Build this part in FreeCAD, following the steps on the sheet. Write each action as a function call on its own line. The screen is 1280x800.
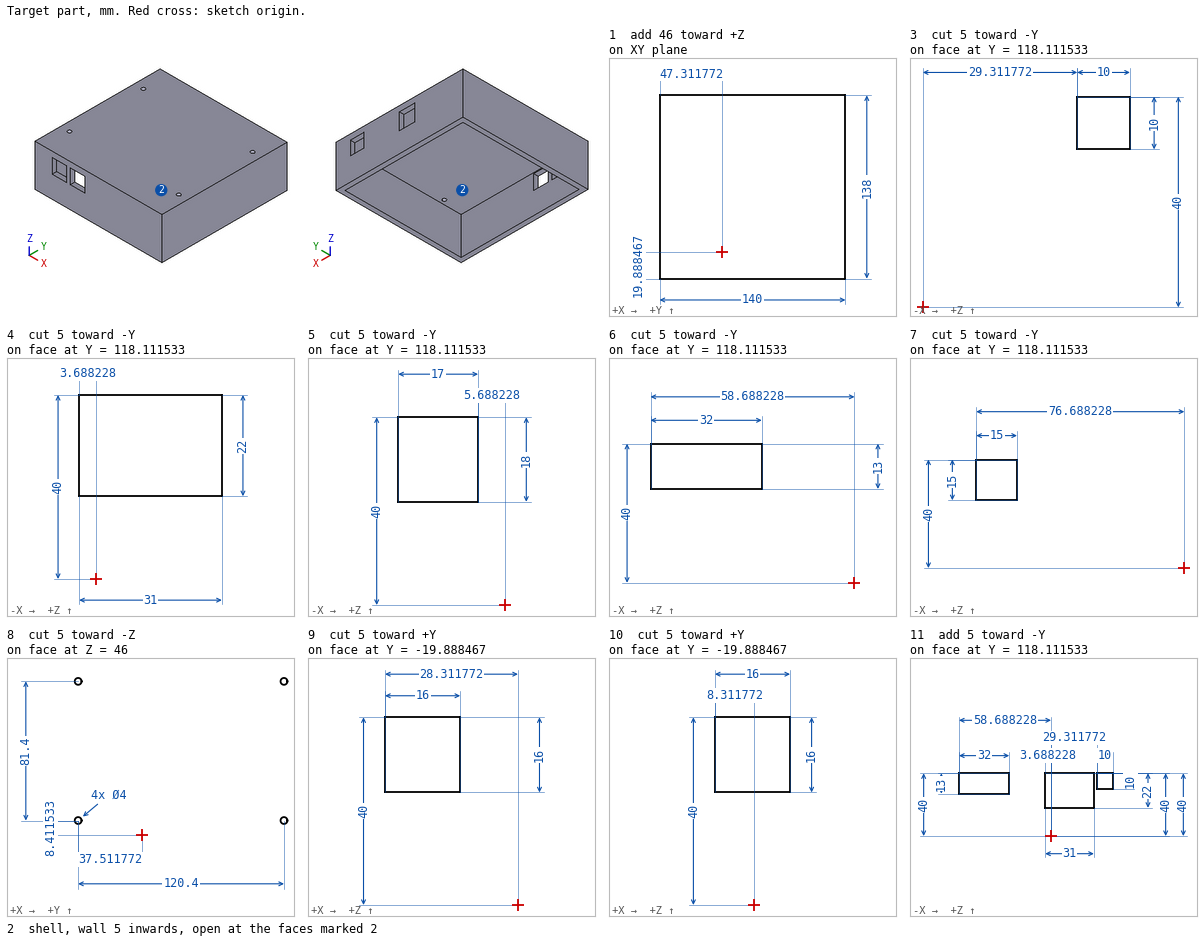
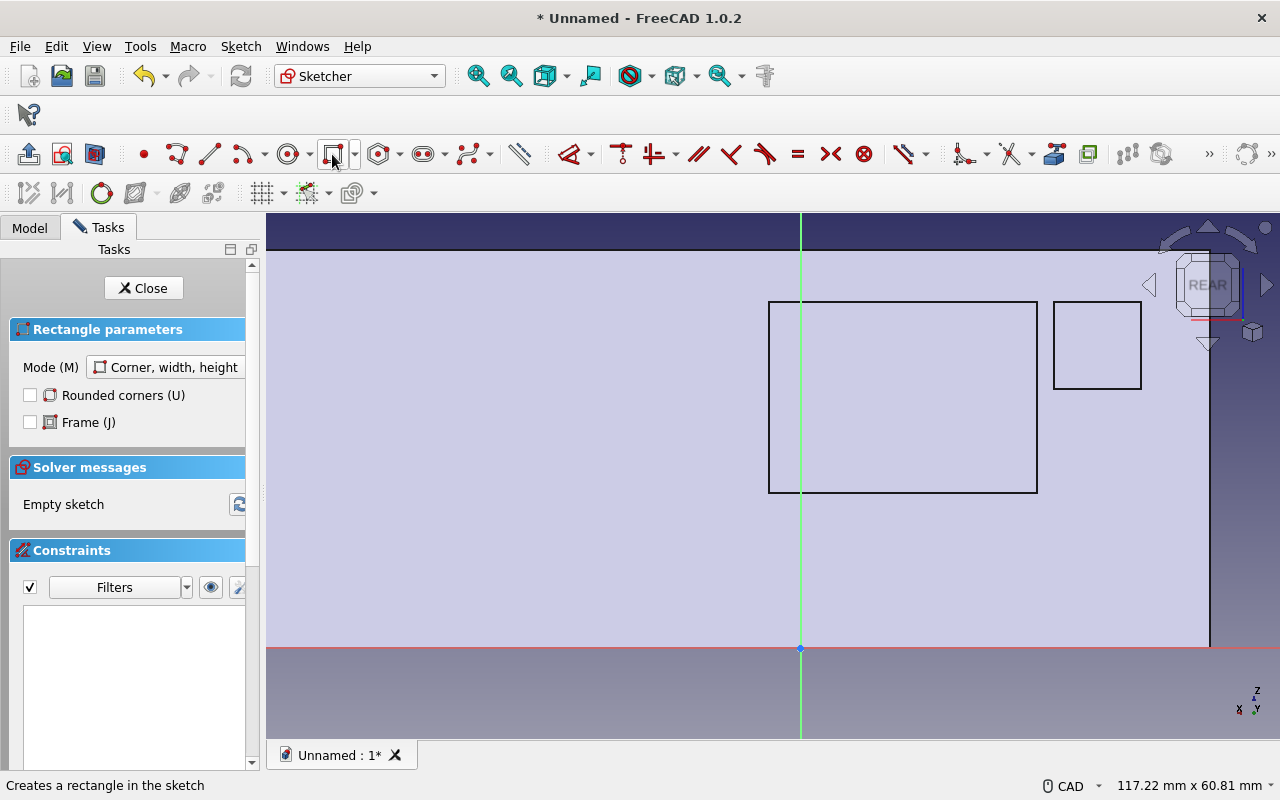
click(605, 302)
move(752, 458)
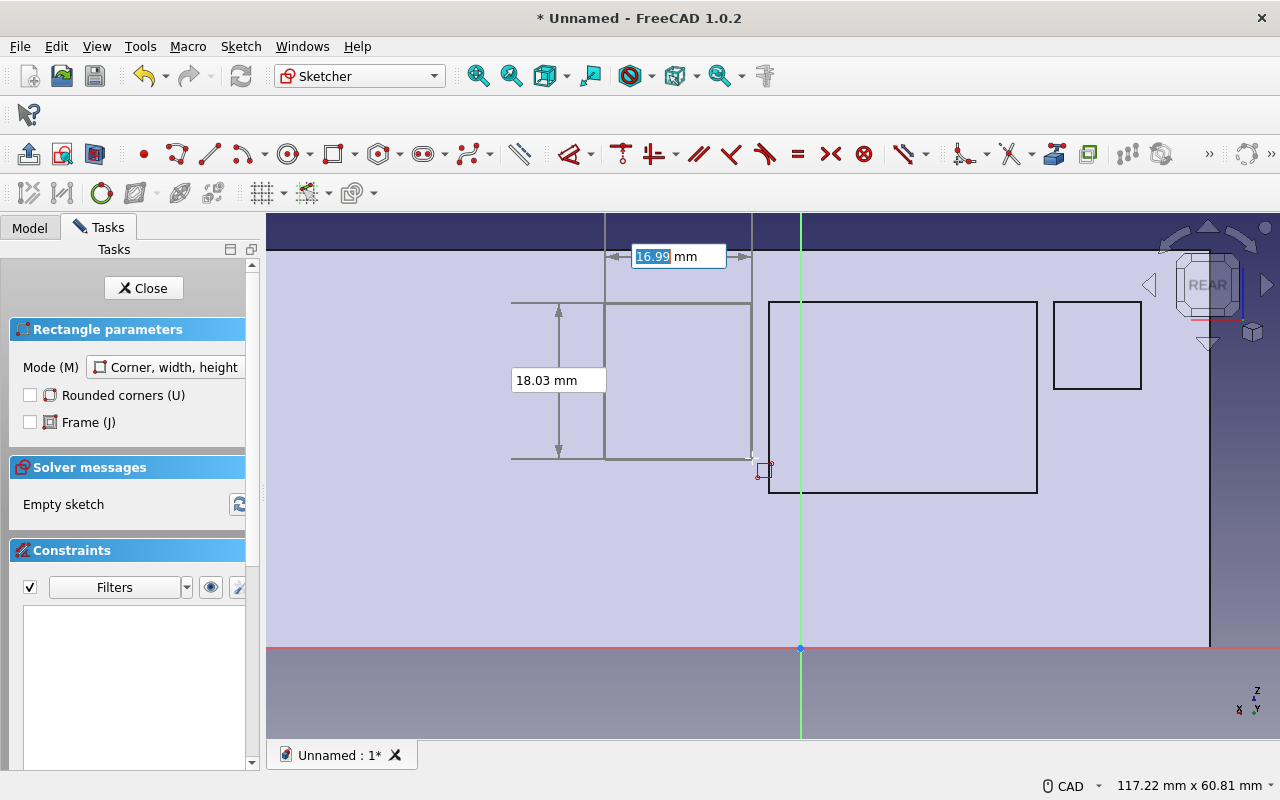
text(17)
key(Tab)
text(18)
key(Return)
key(Escape)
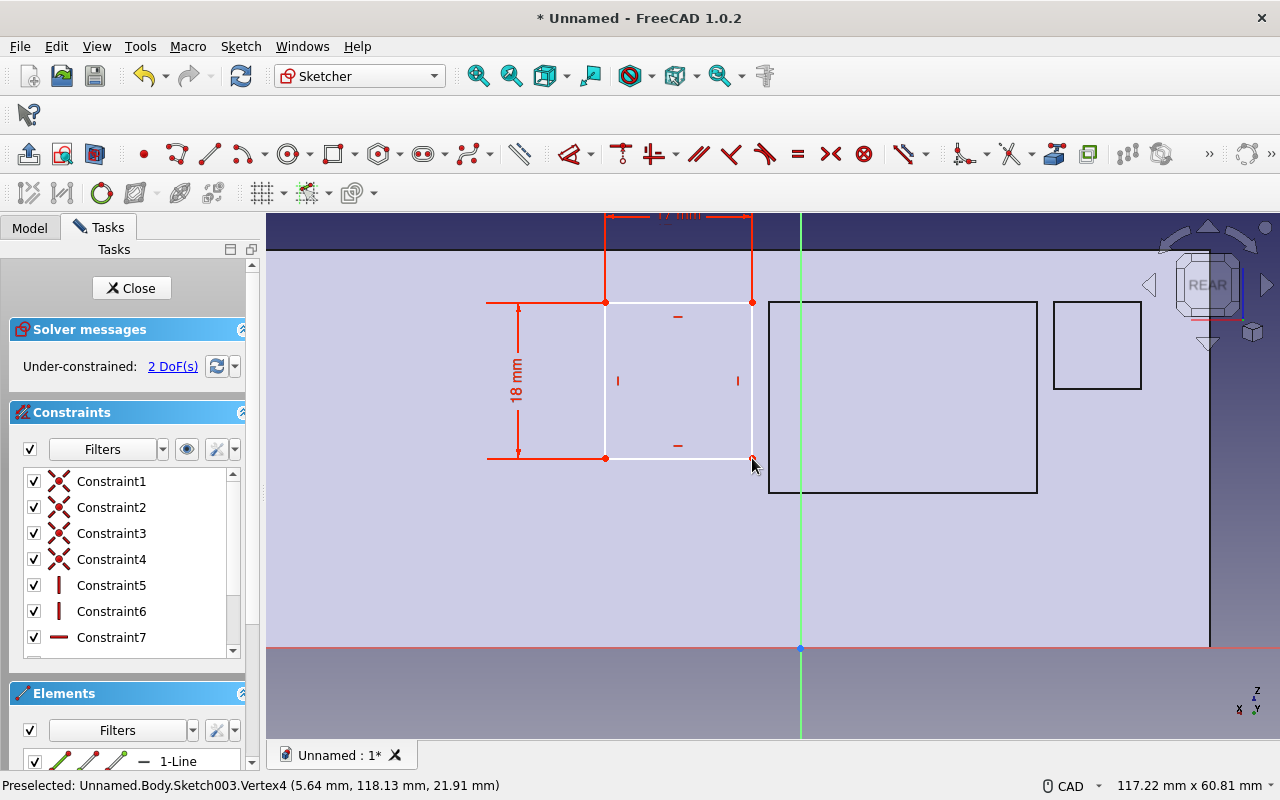
key(d)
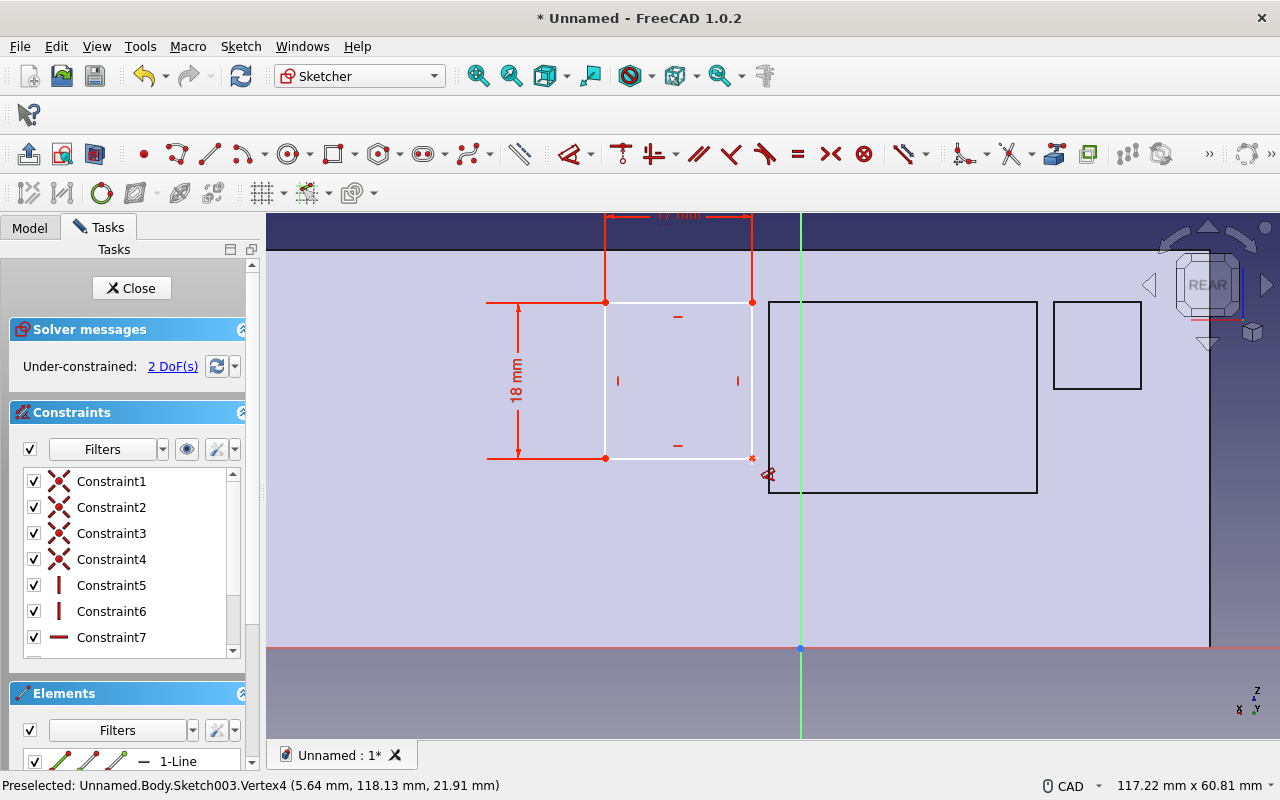
click(605, 303)
click(835, 476)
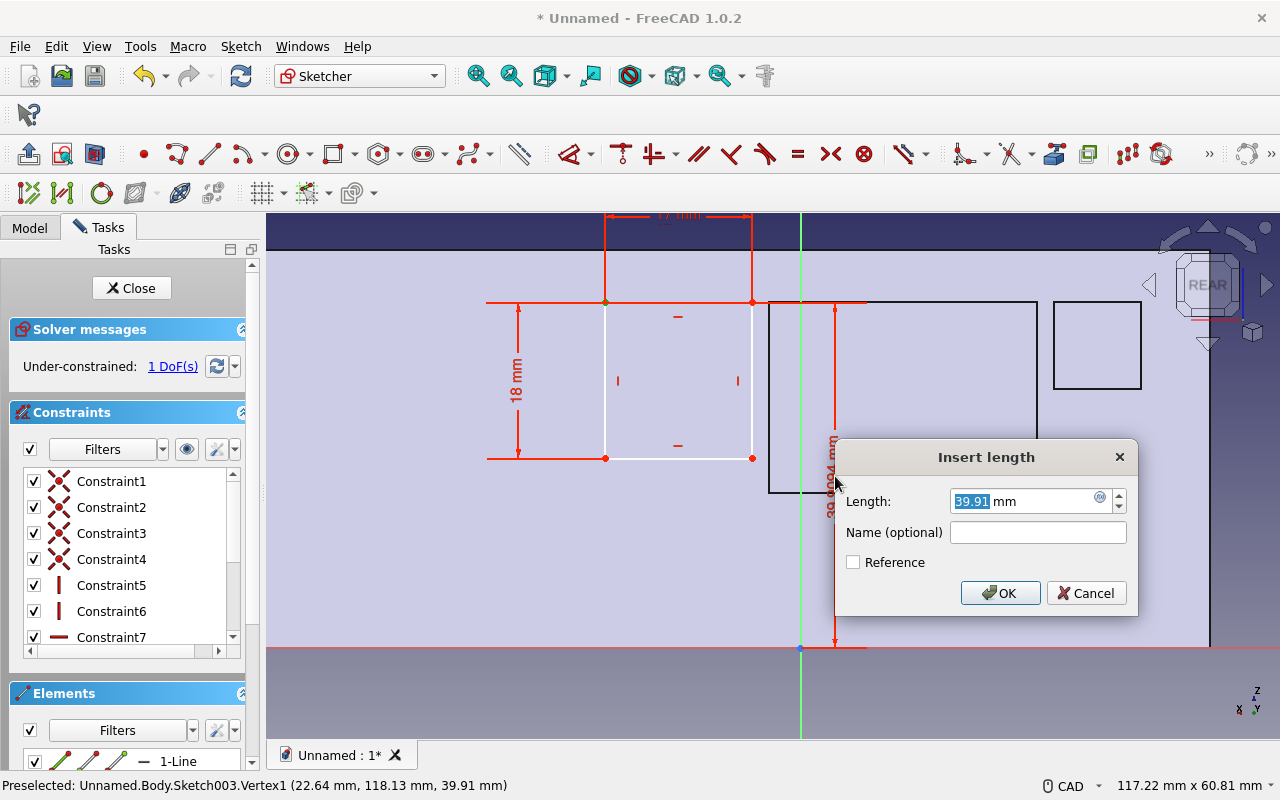
text(40)
key(Return)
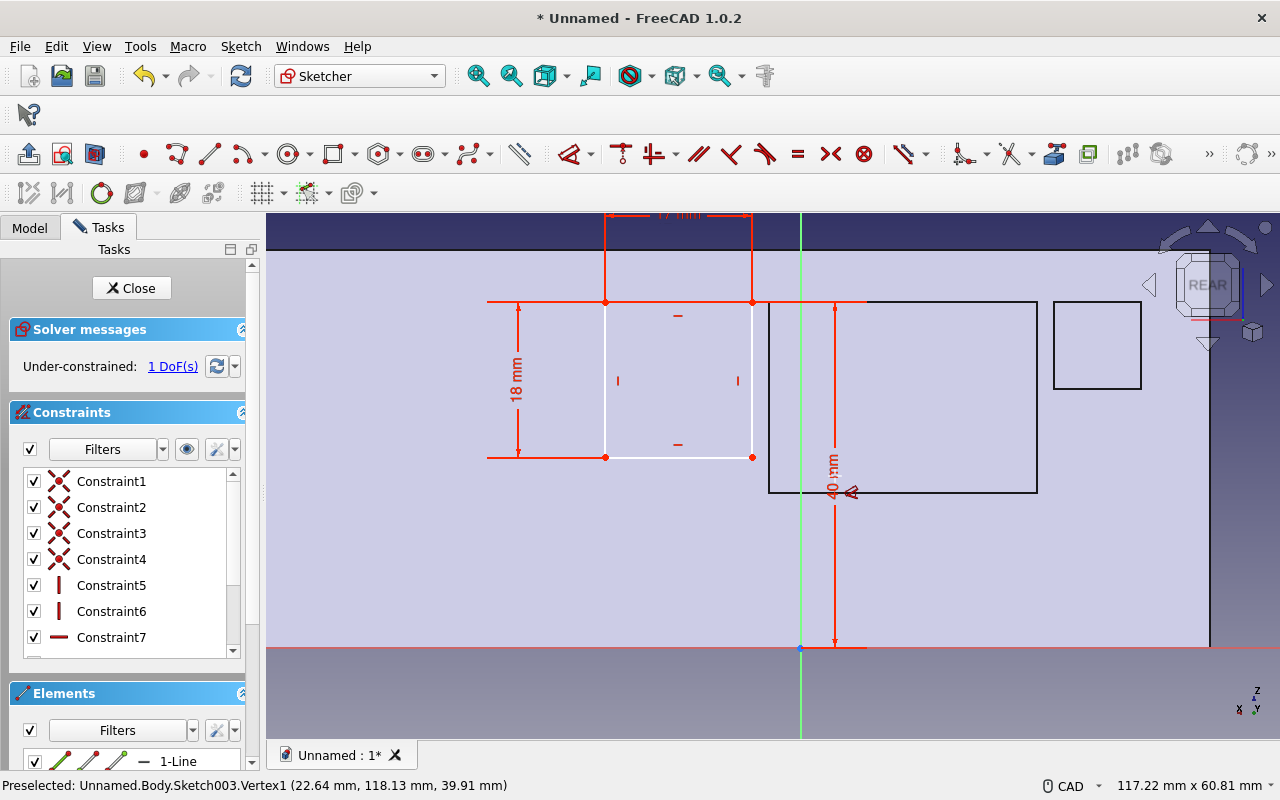
click(752, 458)
click(776, 682)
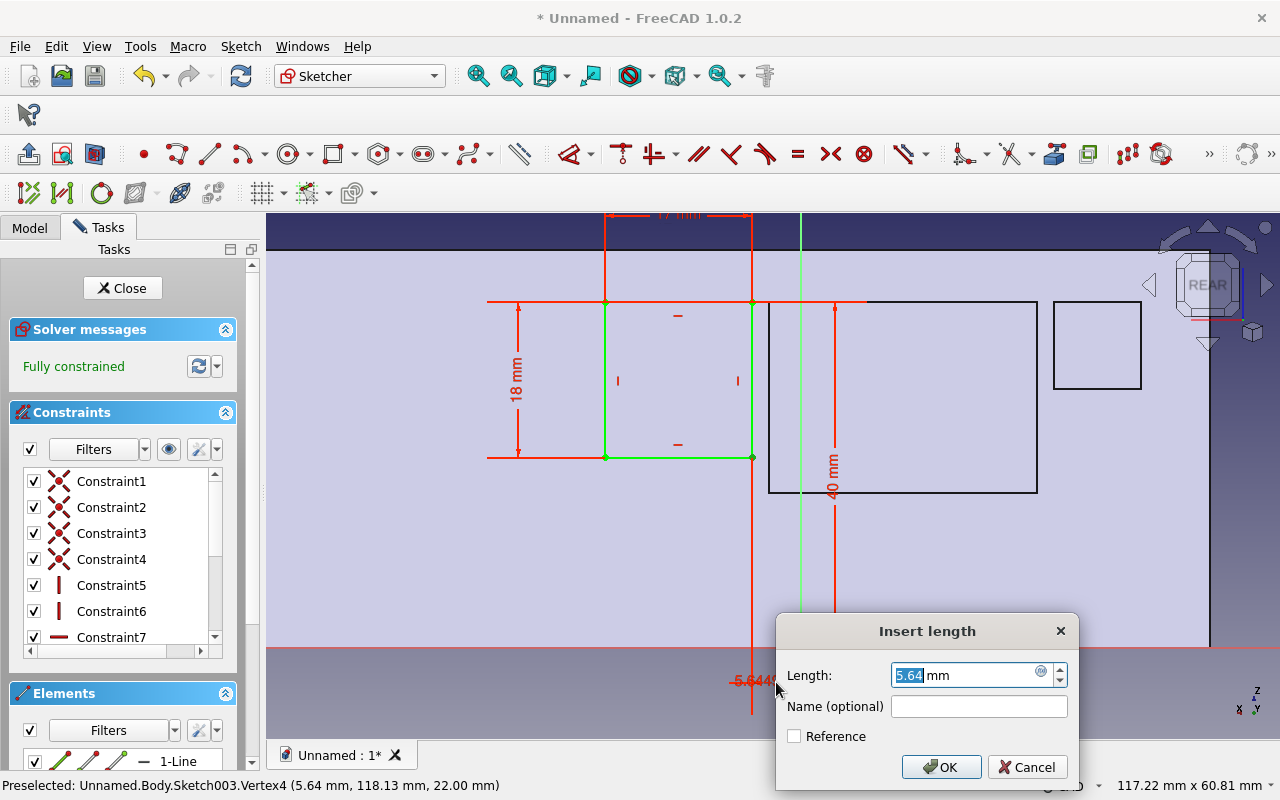
text(5.688228)
key(Return)
key(Escape)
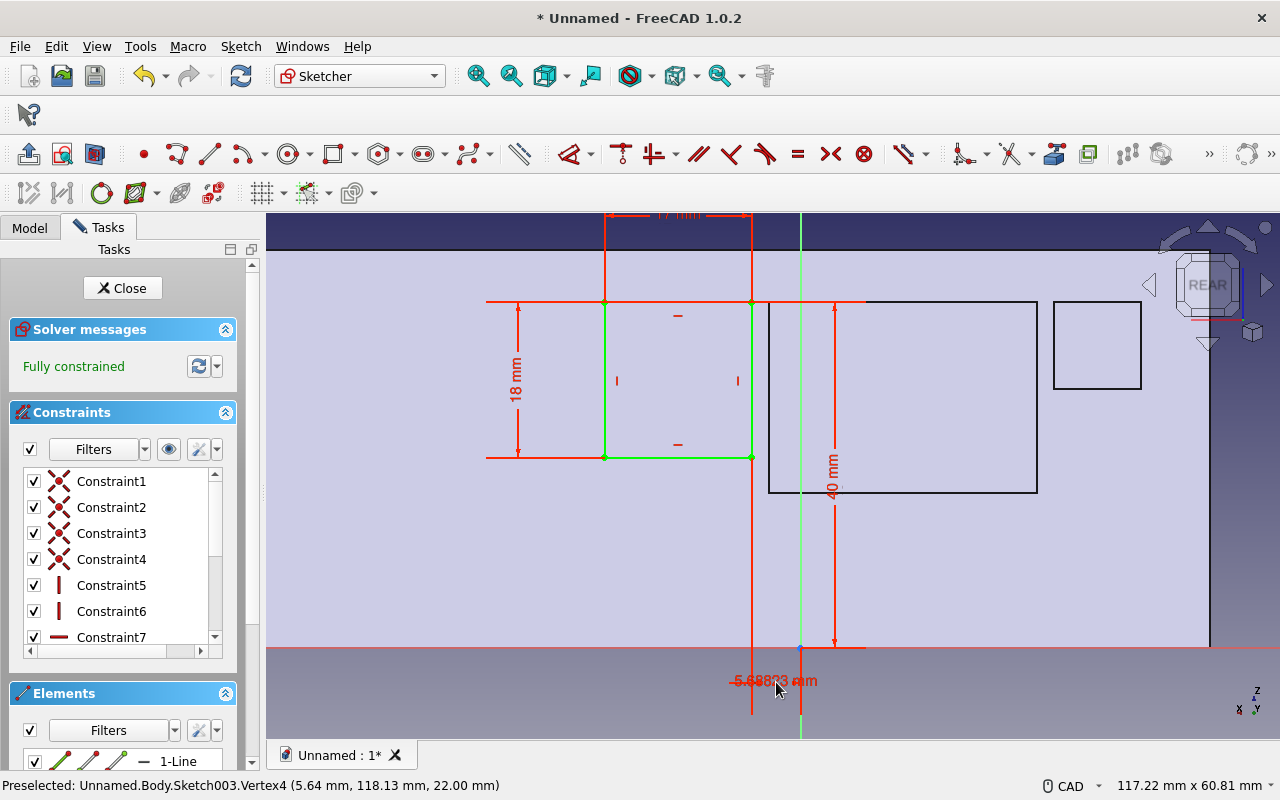
click(123, 288)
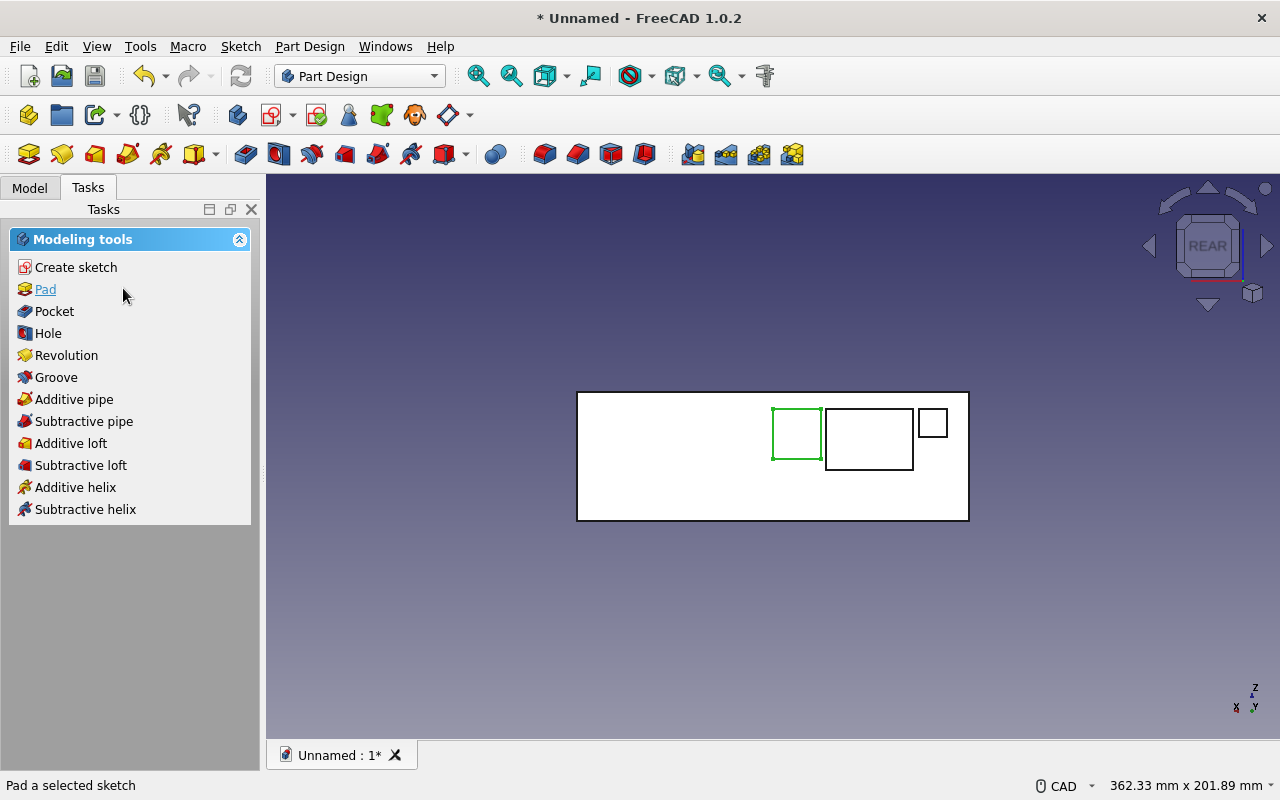
click(246, 154)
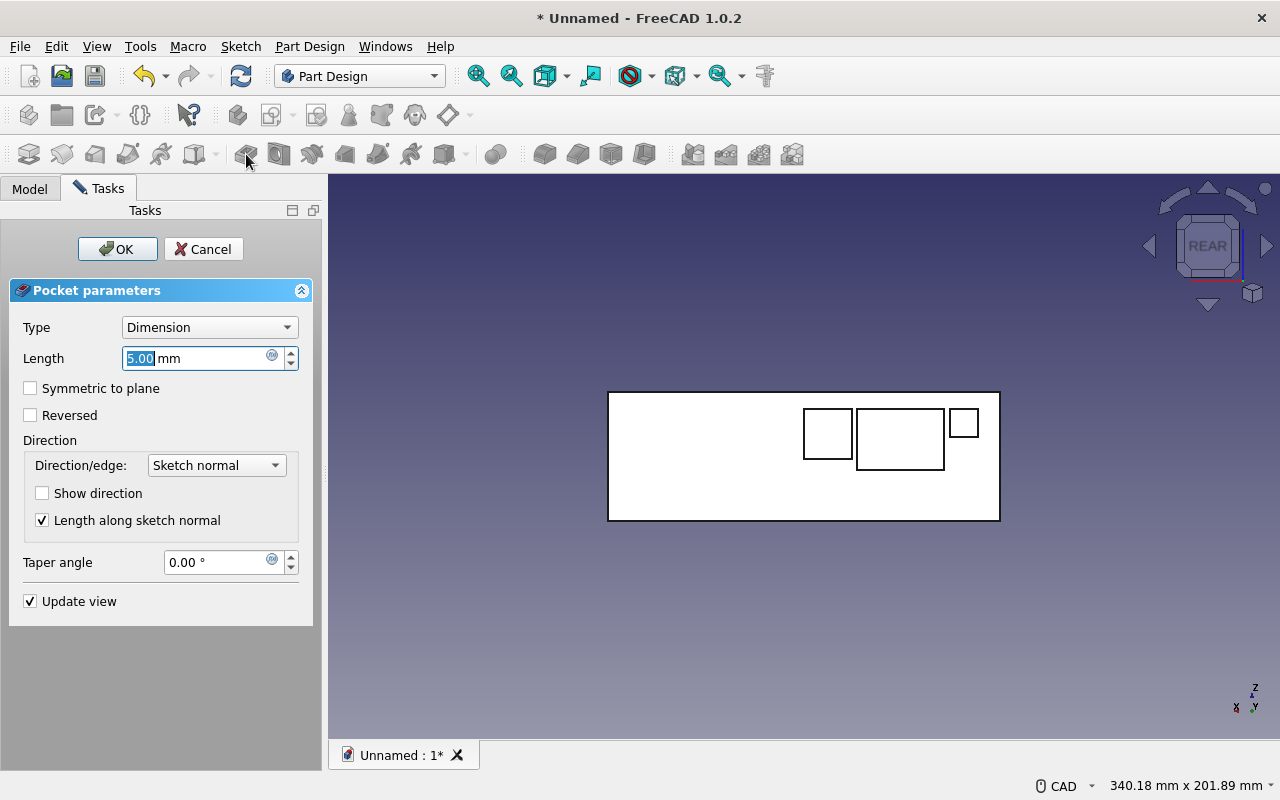
text(5)
key(Tab)